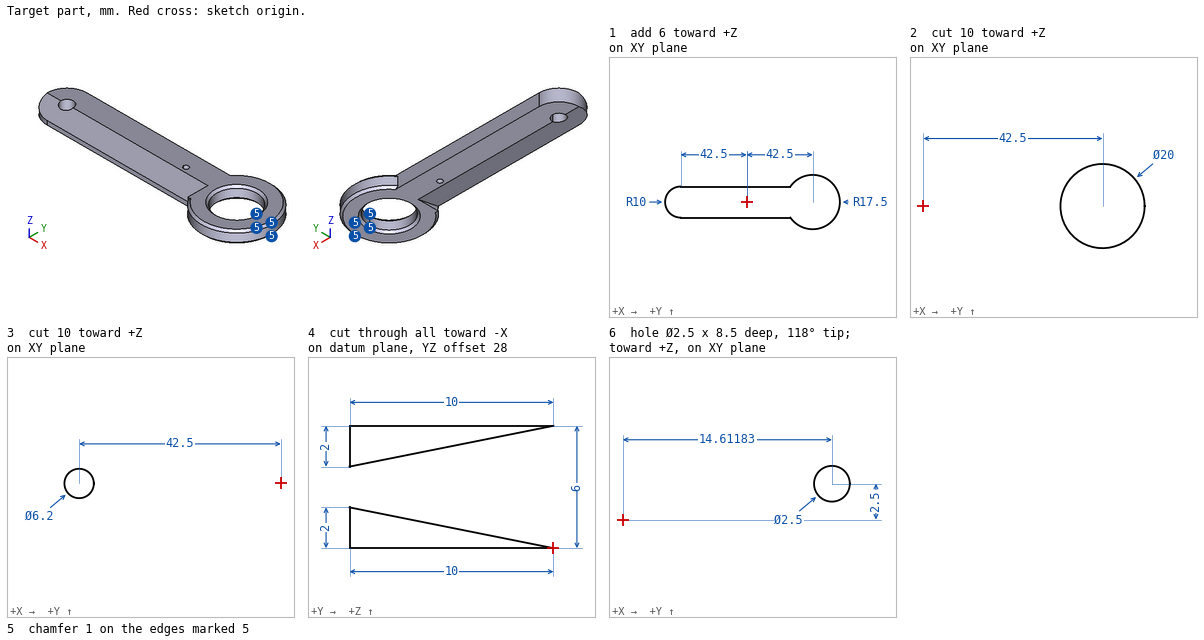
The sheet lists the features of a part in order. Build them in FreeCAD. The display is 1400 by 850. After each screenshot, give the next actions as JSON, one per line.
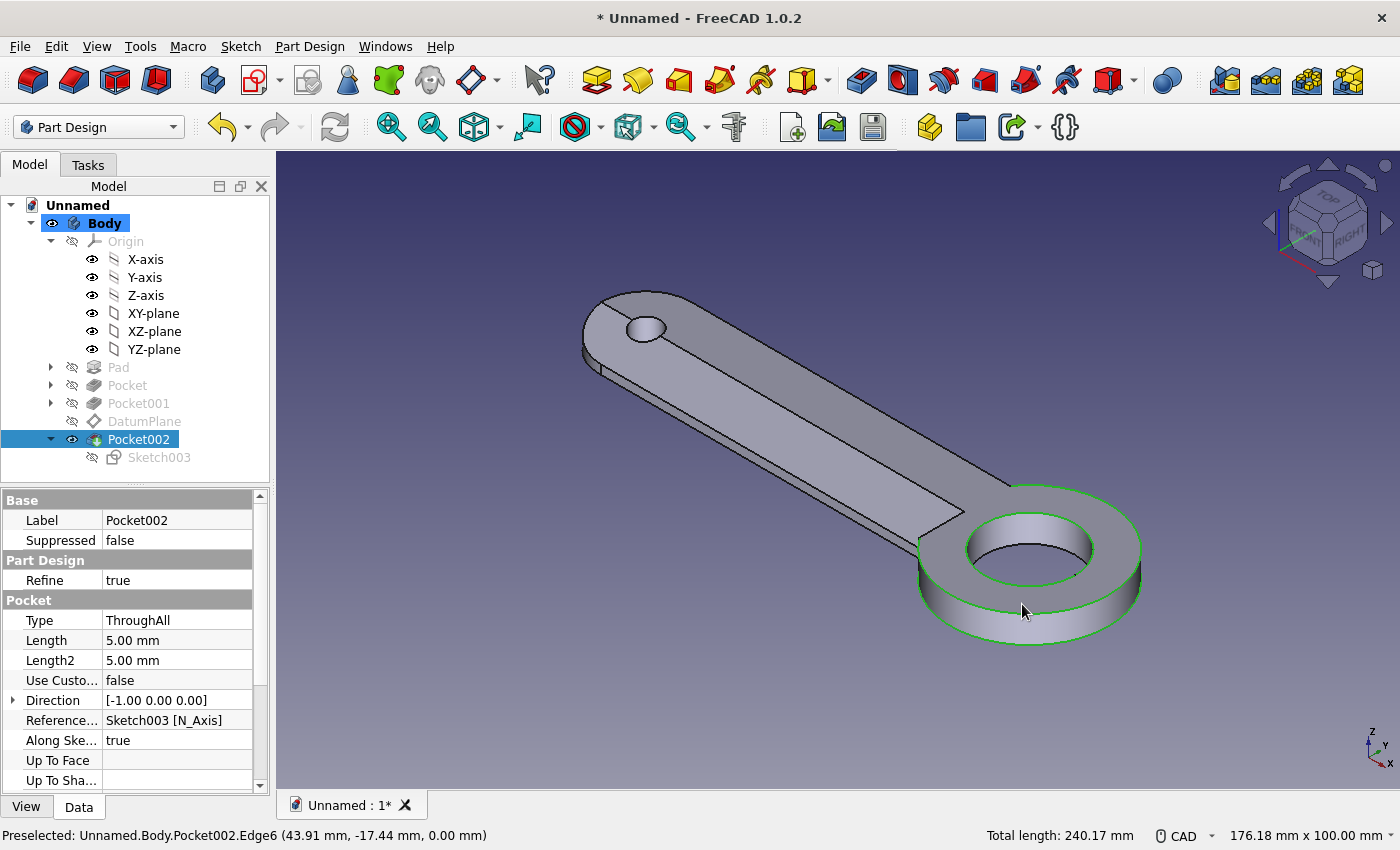
{"action": "key", "text": "2"}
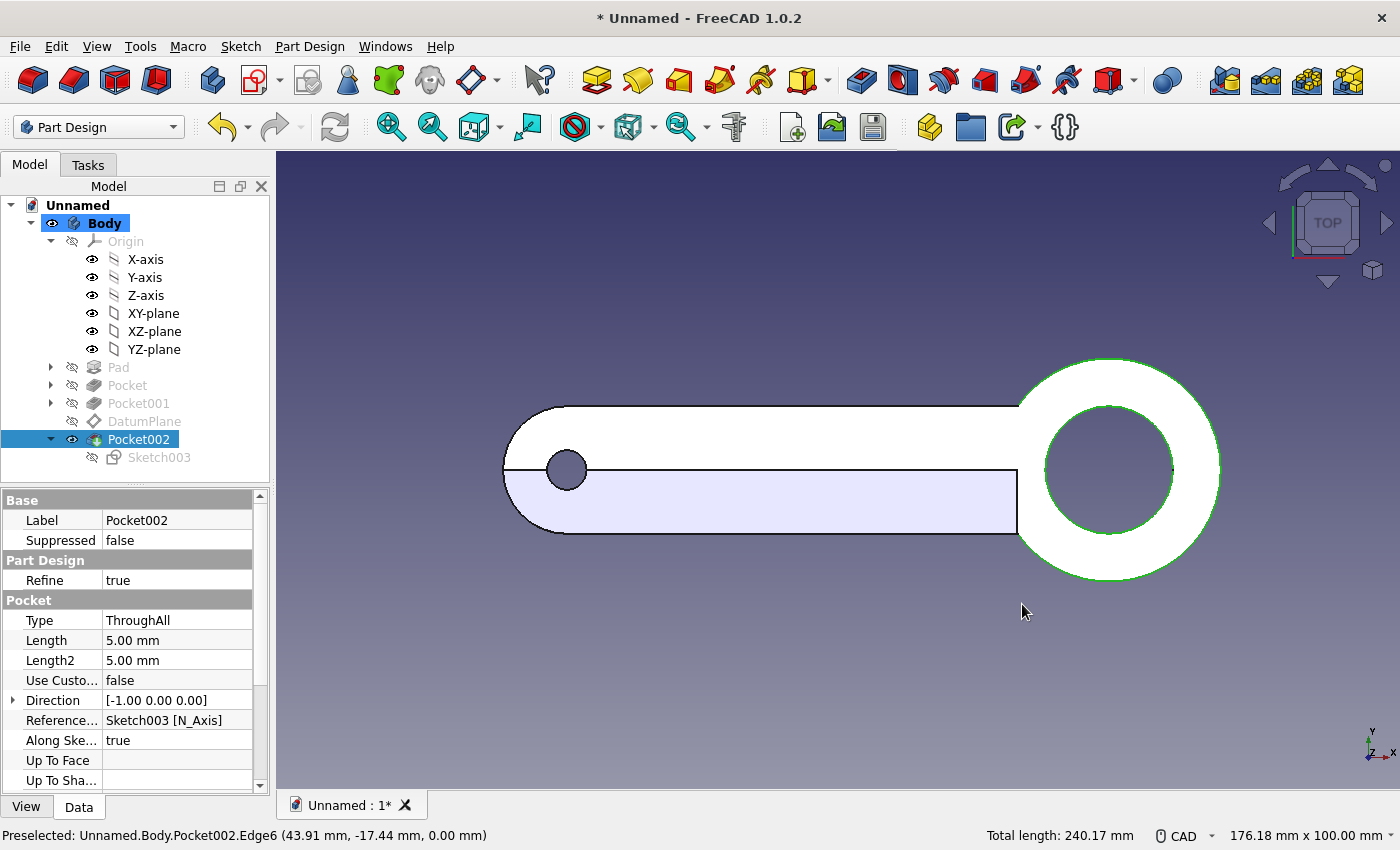
{"action": "key", "text": "1"}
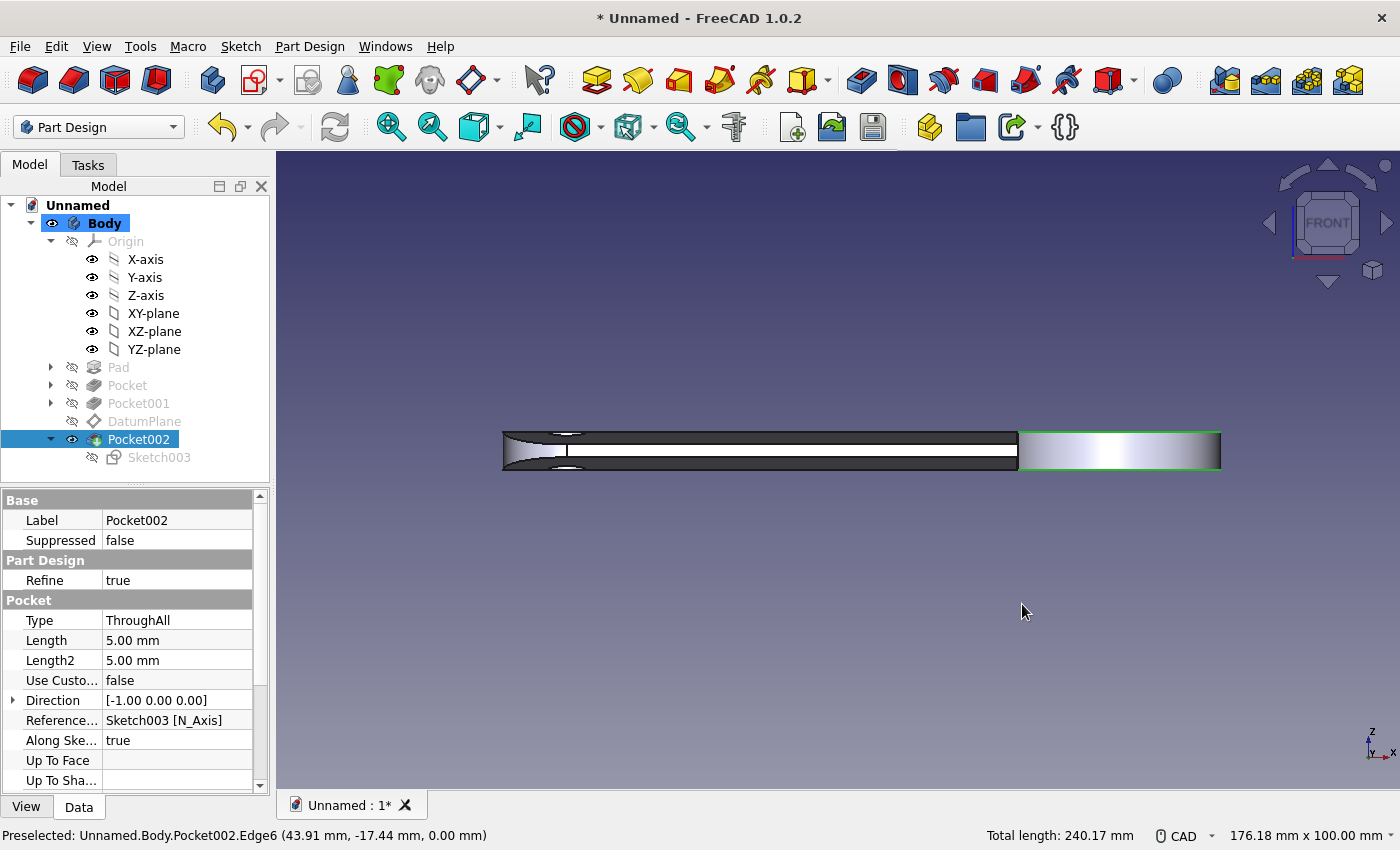
{"action": "key", "text": "3"}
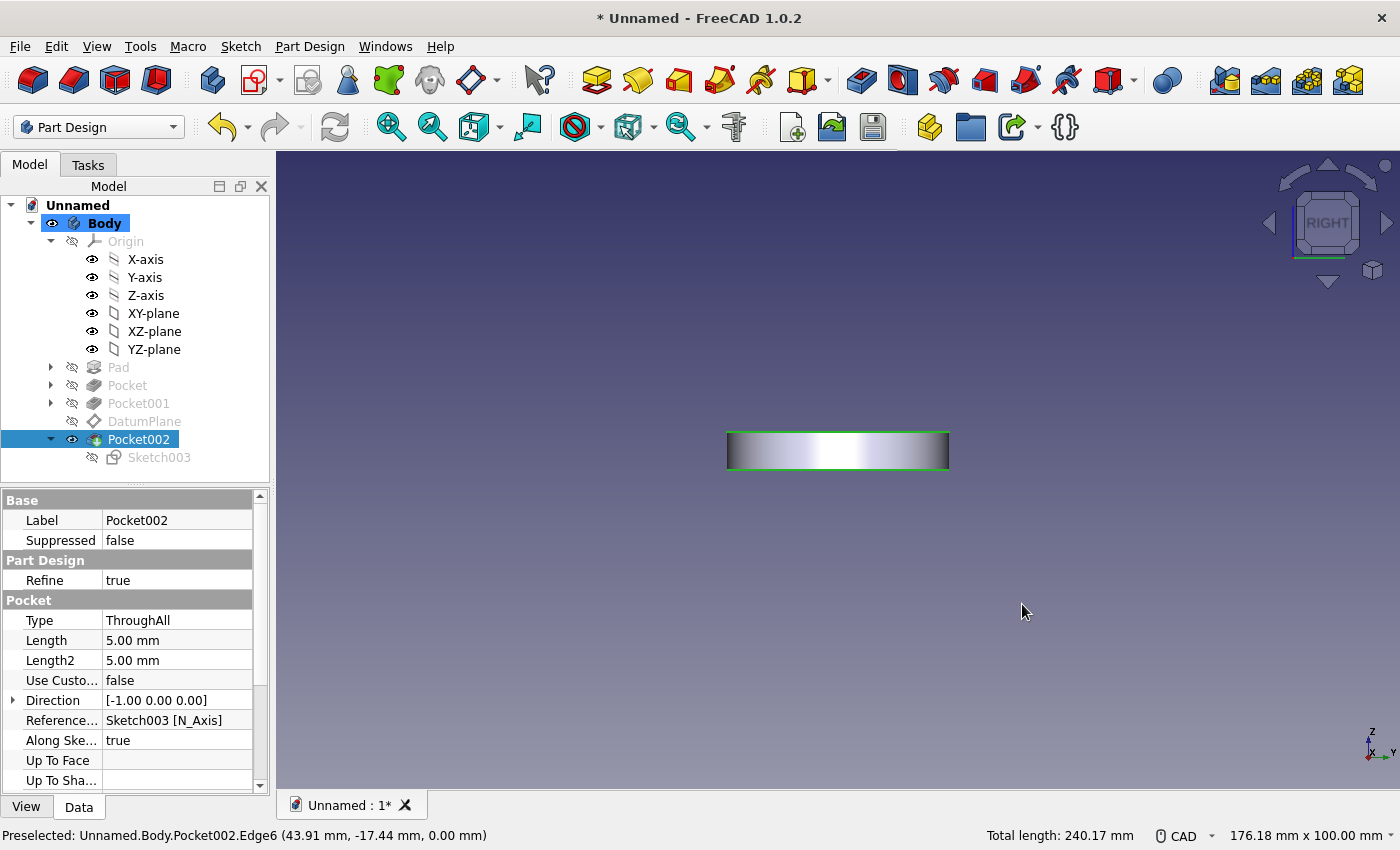
{"action": "key", "text": "v f"}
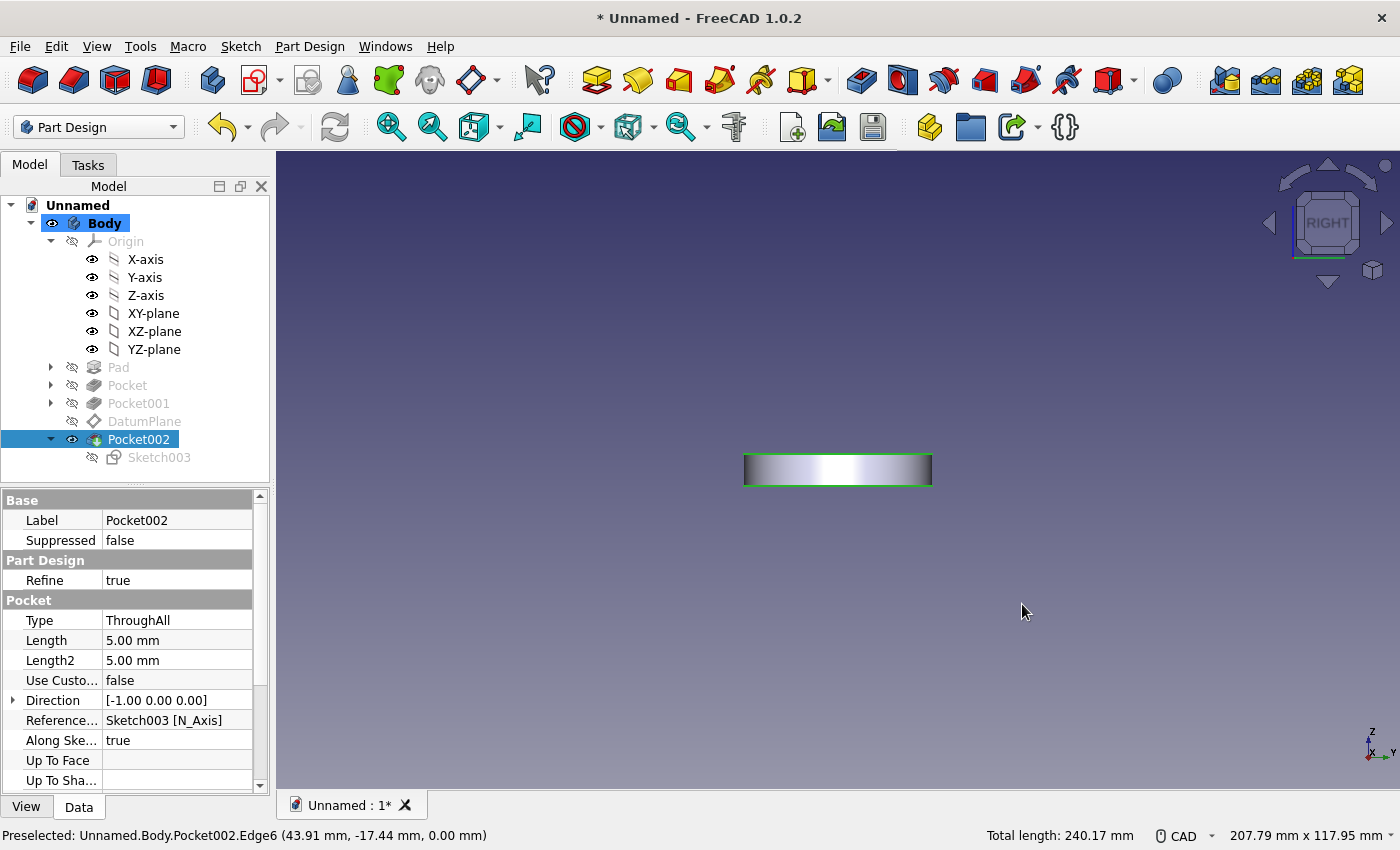
{"action": "key", "text": "5"}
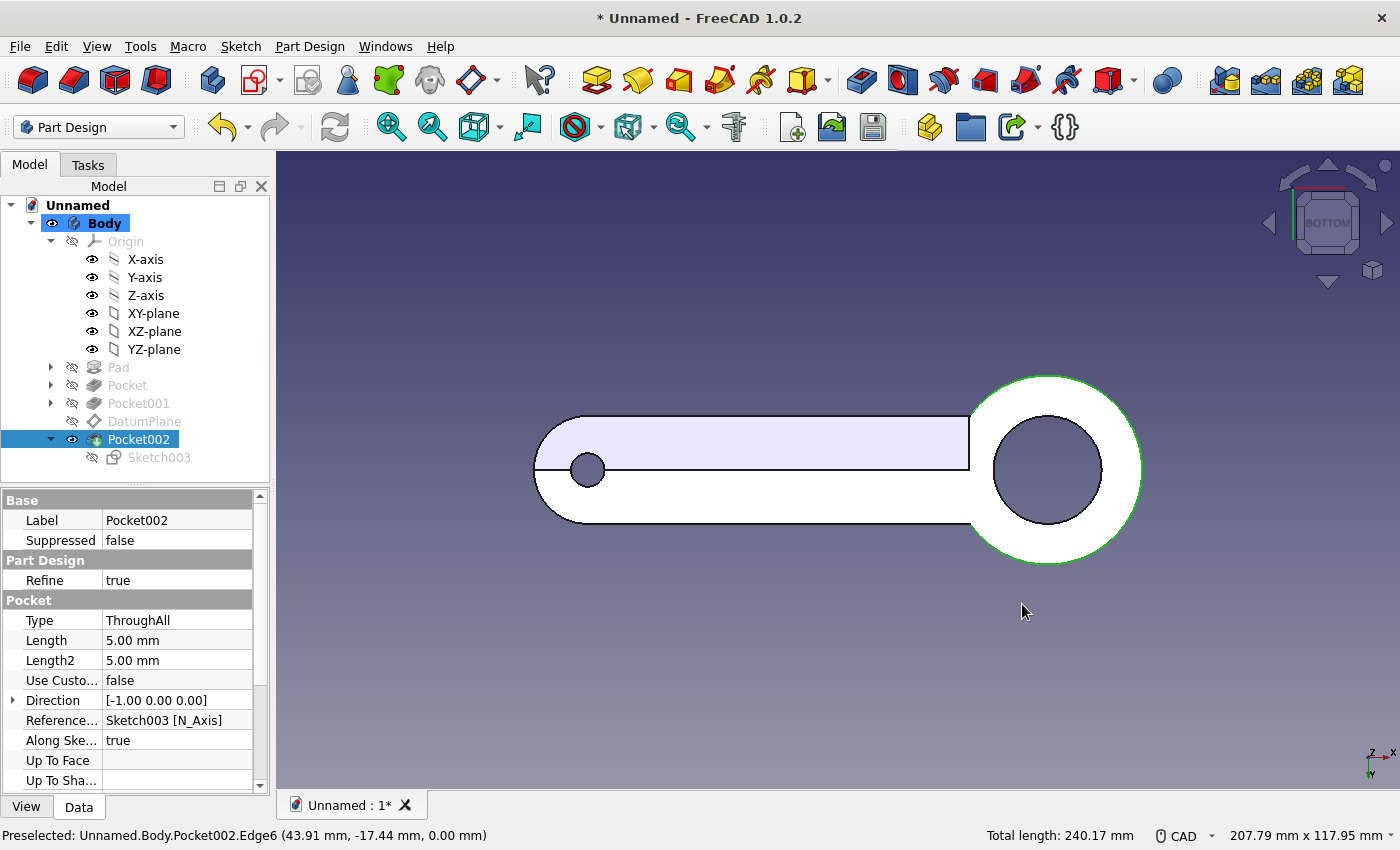
{"action": "left_click", "coordinate": [994, 469], "text": "ctrl"}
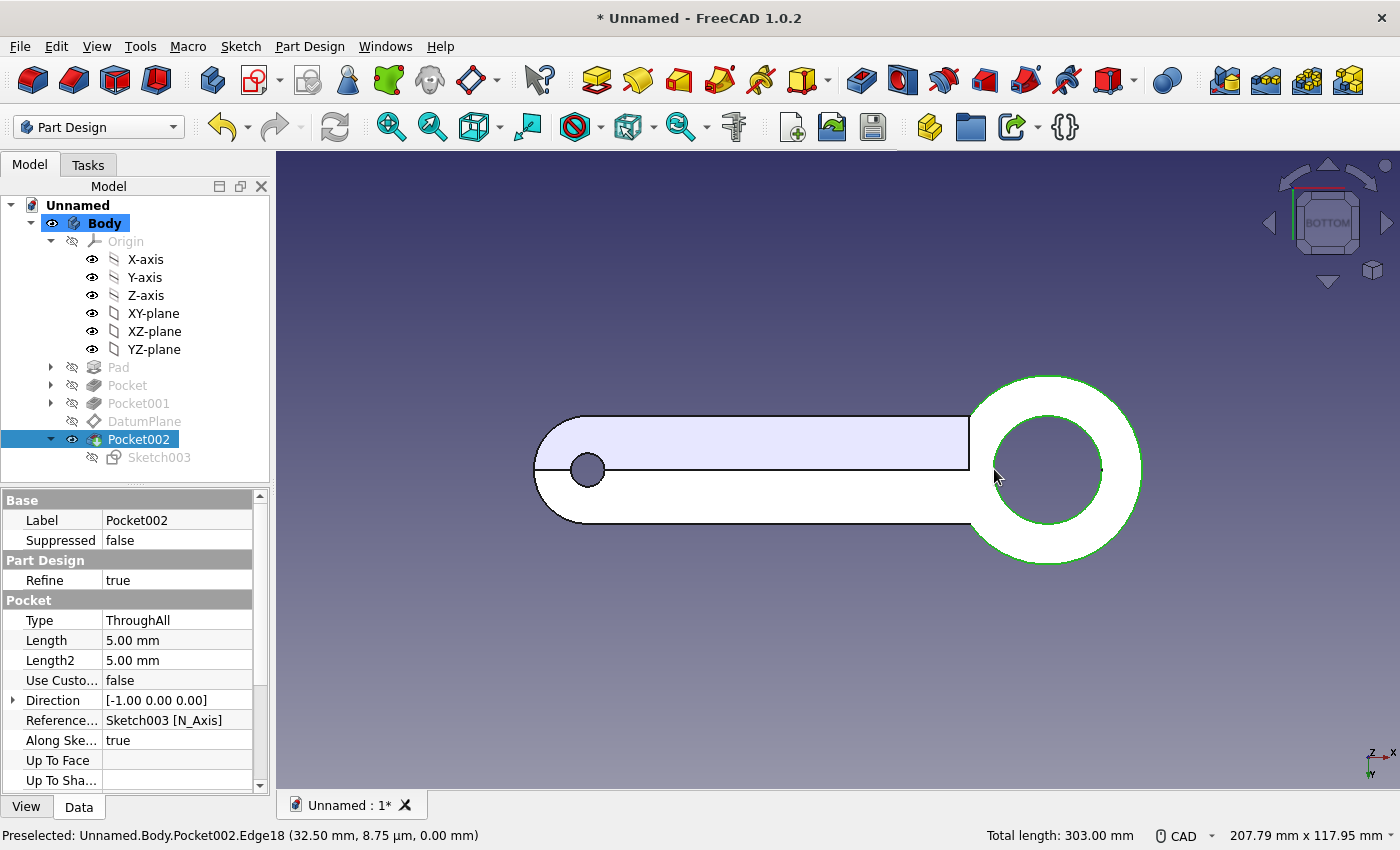
{"action": "left_click", "coordinate": [74, 80]}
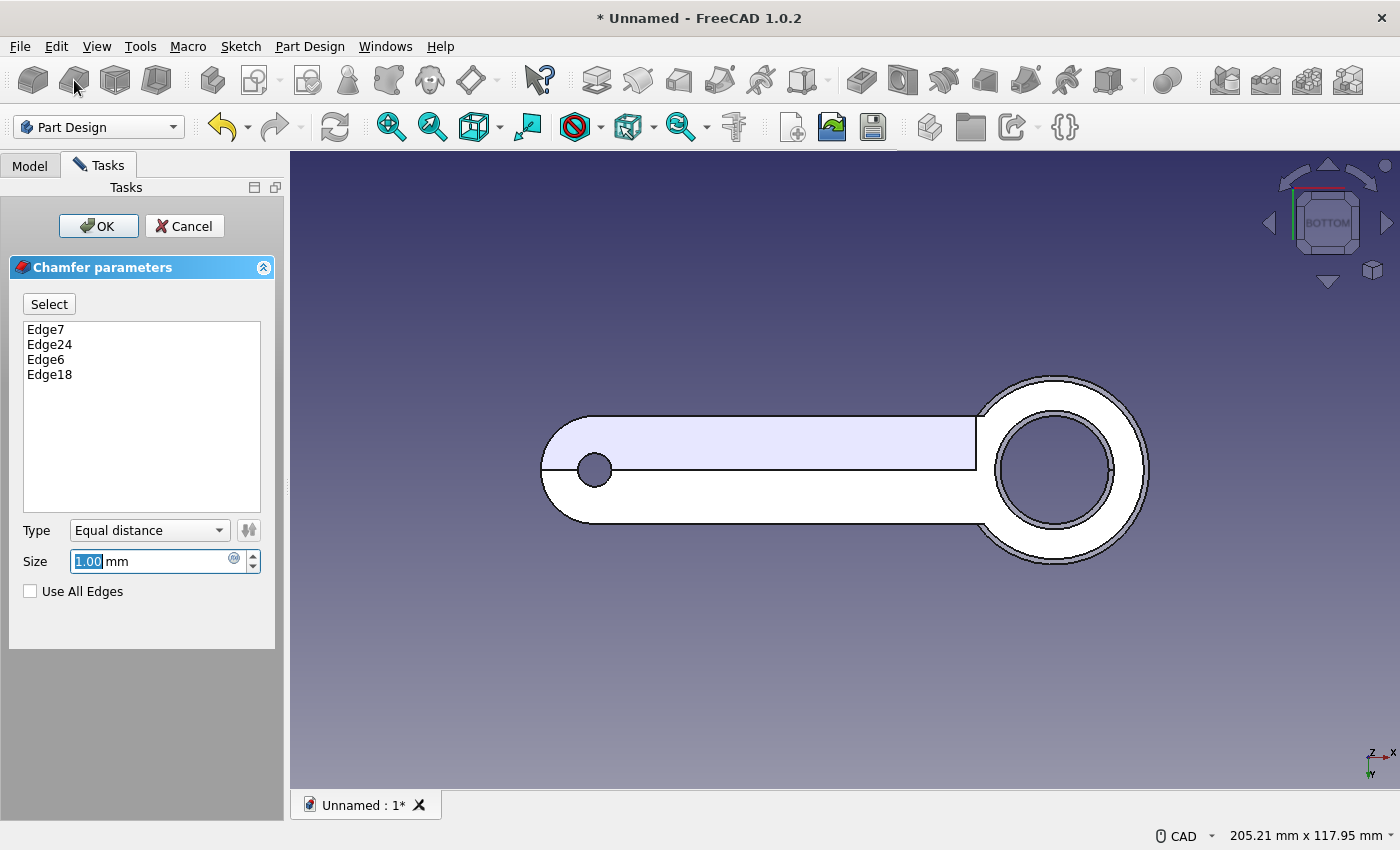
{"action": "type", "text": "1"}
{"action": "key", "text": "Tab"}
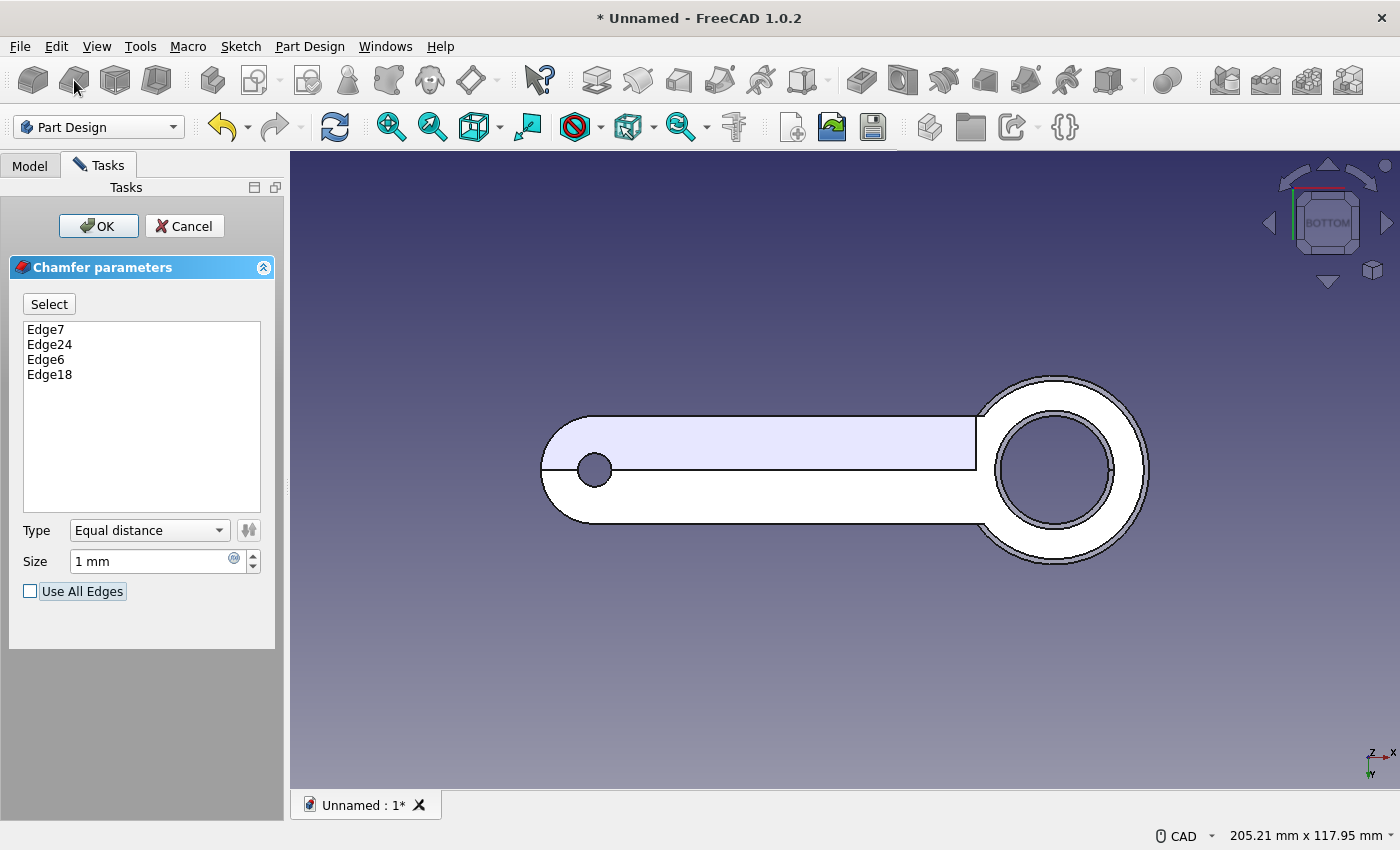
{"action": "left_click", "coordinate": [99, 226]}